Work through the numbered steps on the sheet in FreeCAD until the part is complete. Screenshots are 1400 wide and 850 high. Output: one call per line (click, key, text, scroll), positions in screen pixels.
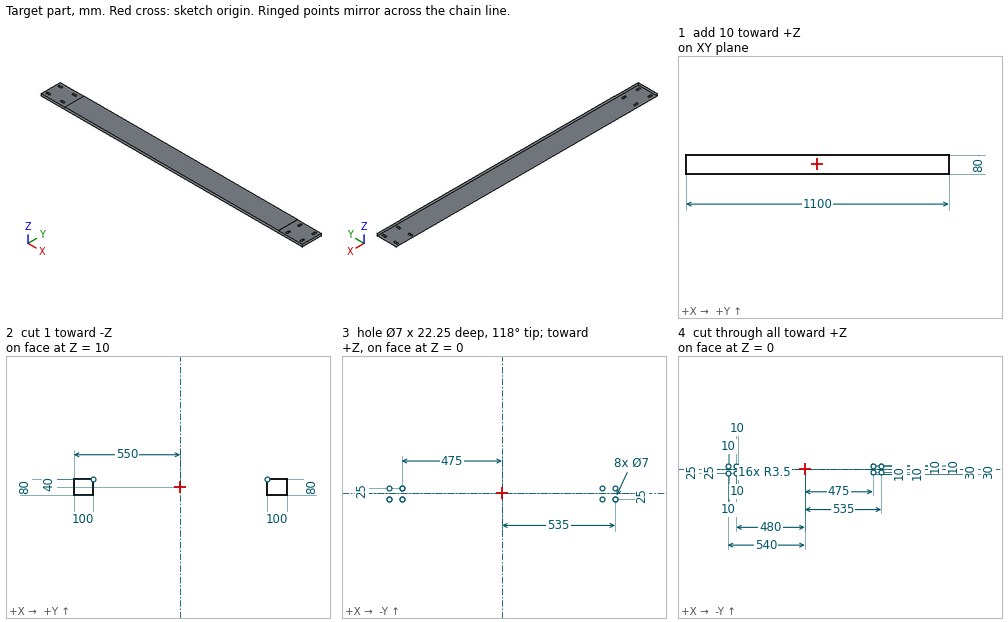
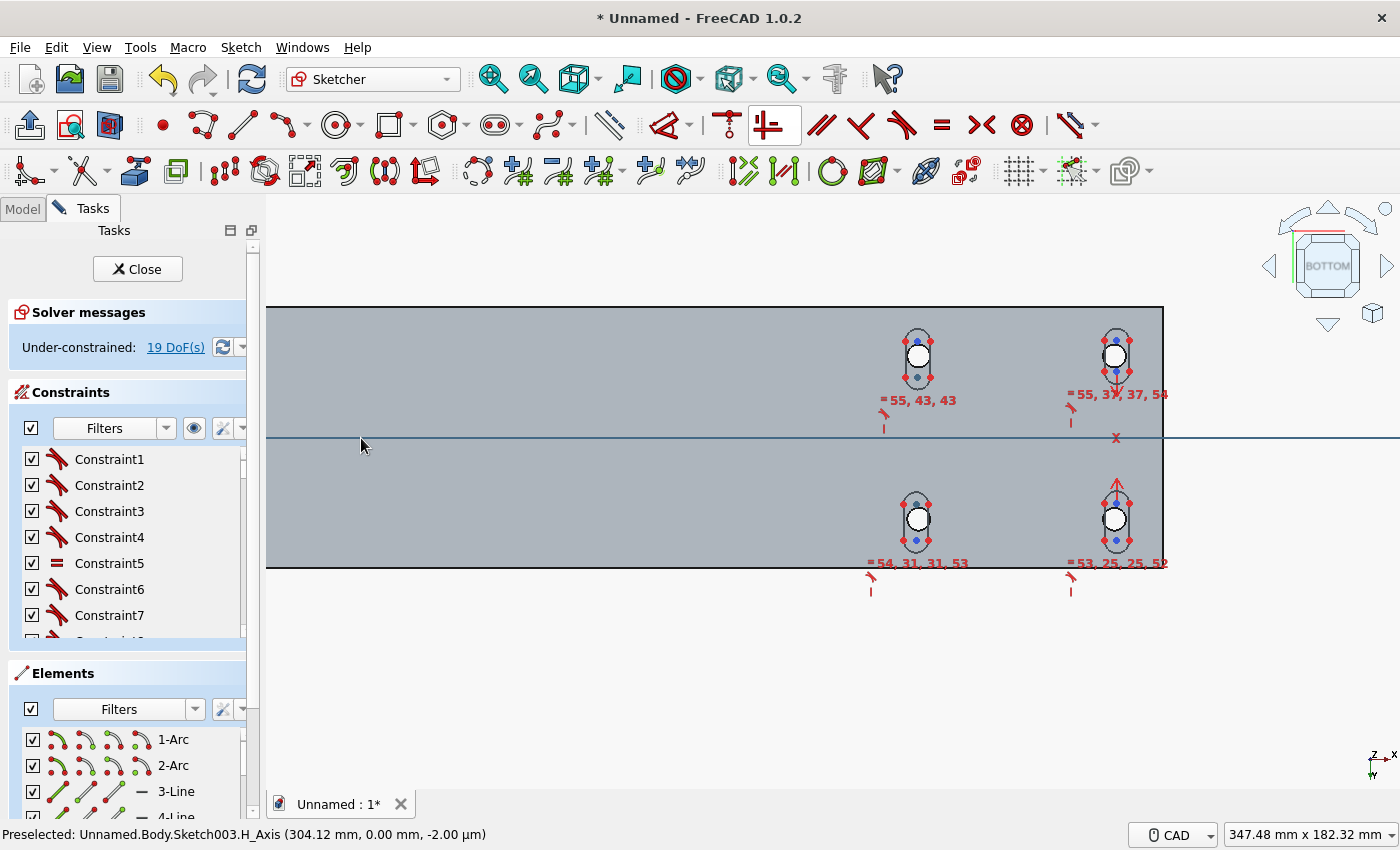
click(982, 126)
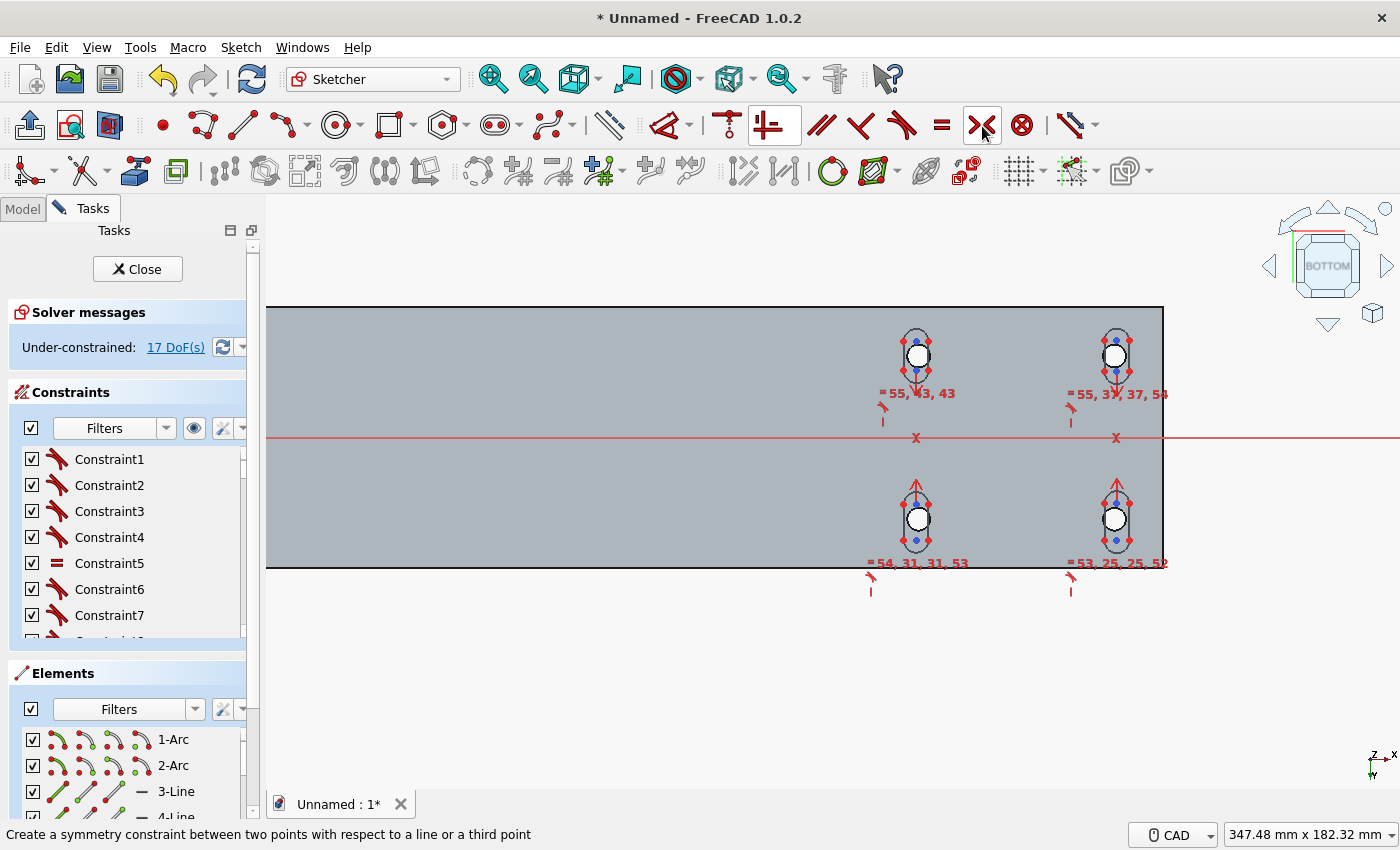
click(664, 126)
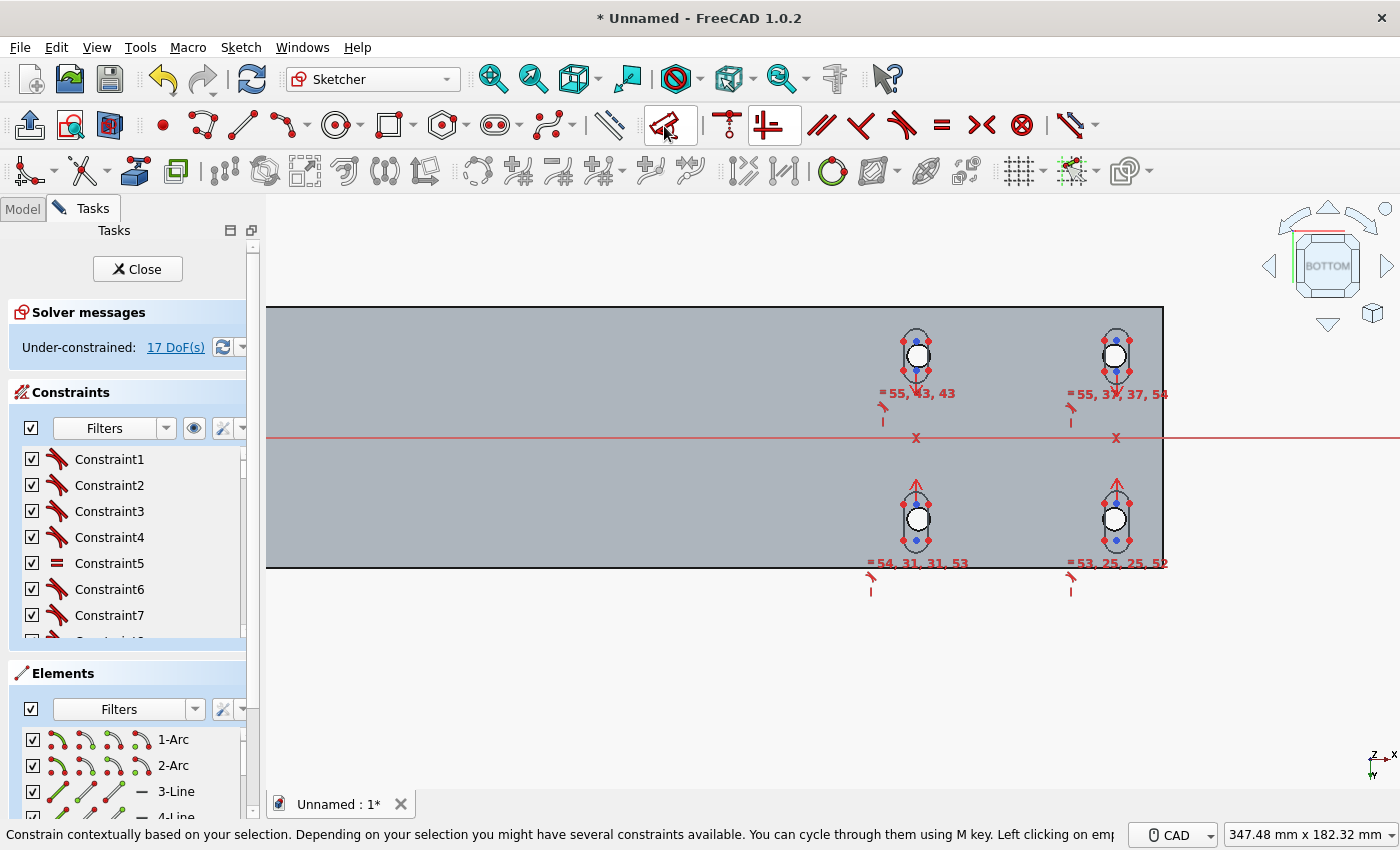
scroll(1120, 505, down, 8)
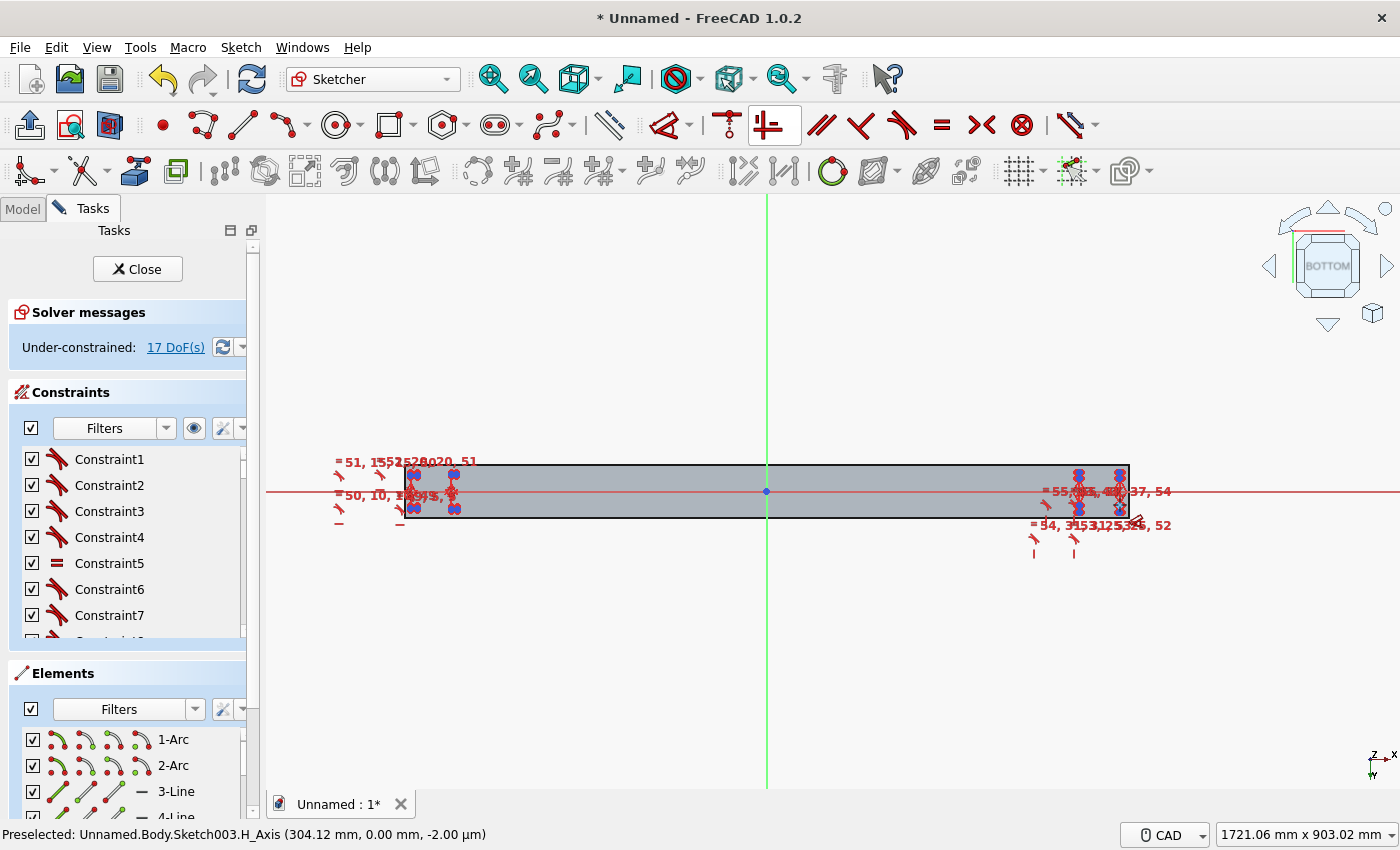
scroll(449, 508, up, 15)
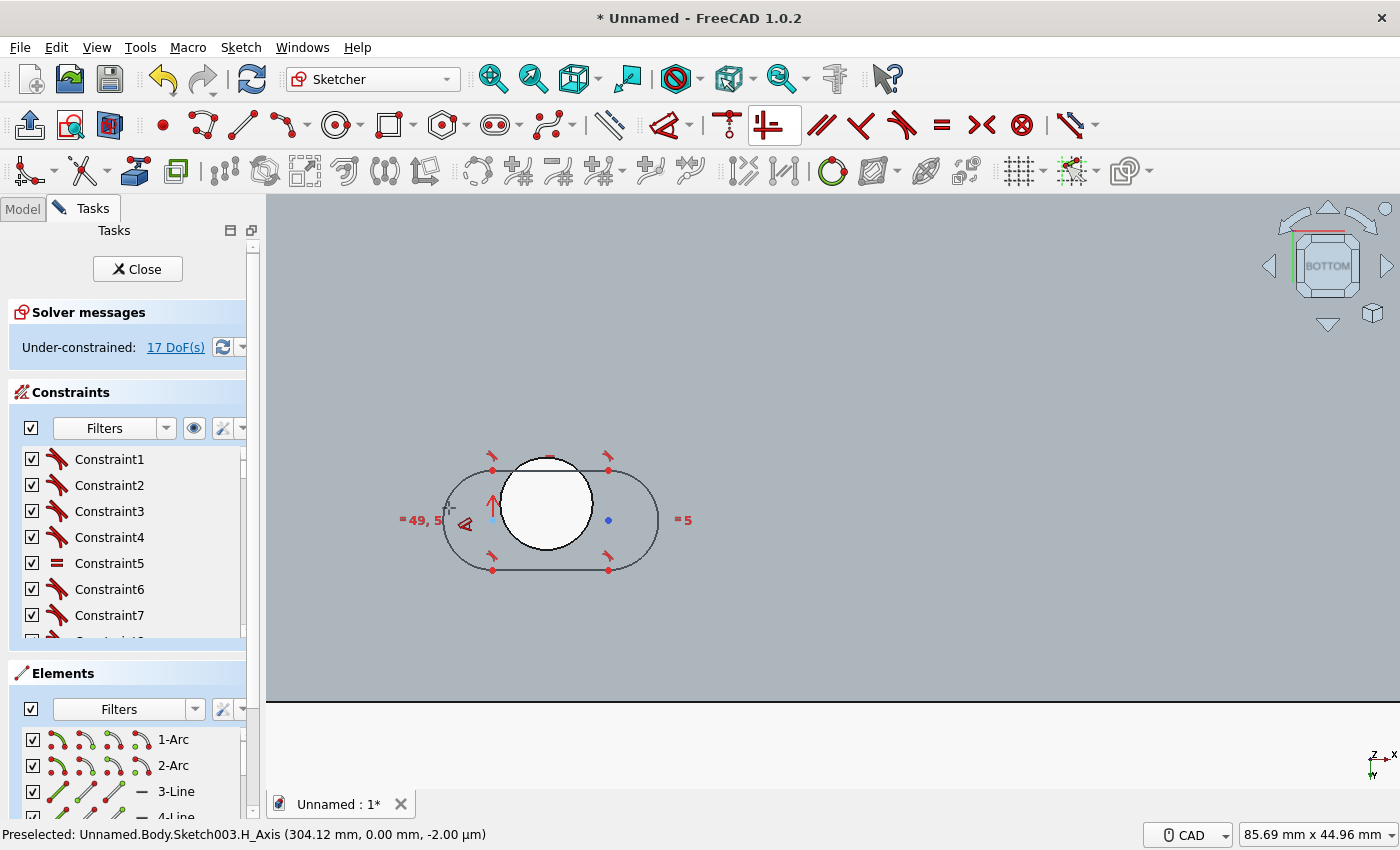
click(453, 491)
click(427, 472)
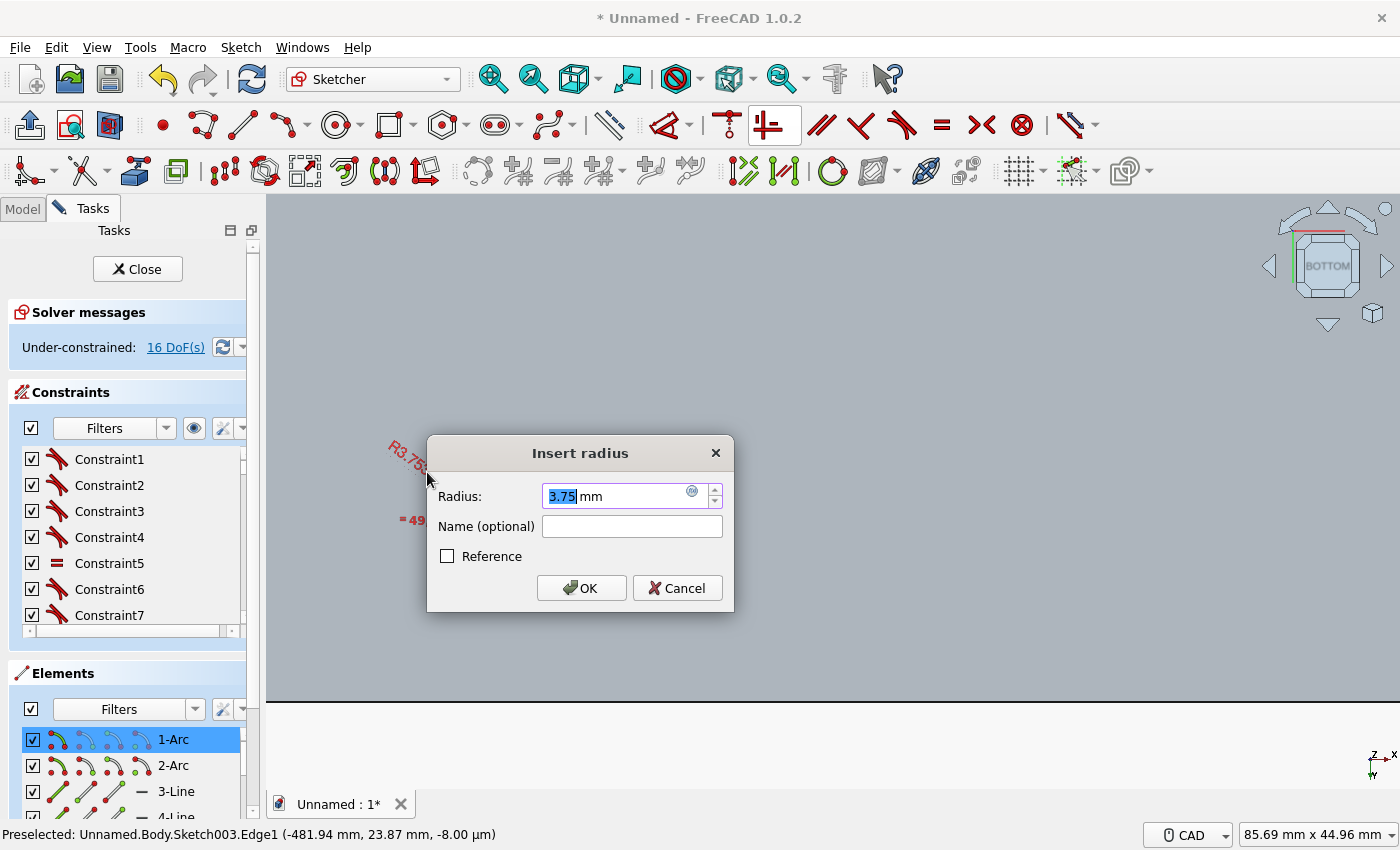
text(3.5)
key(Return)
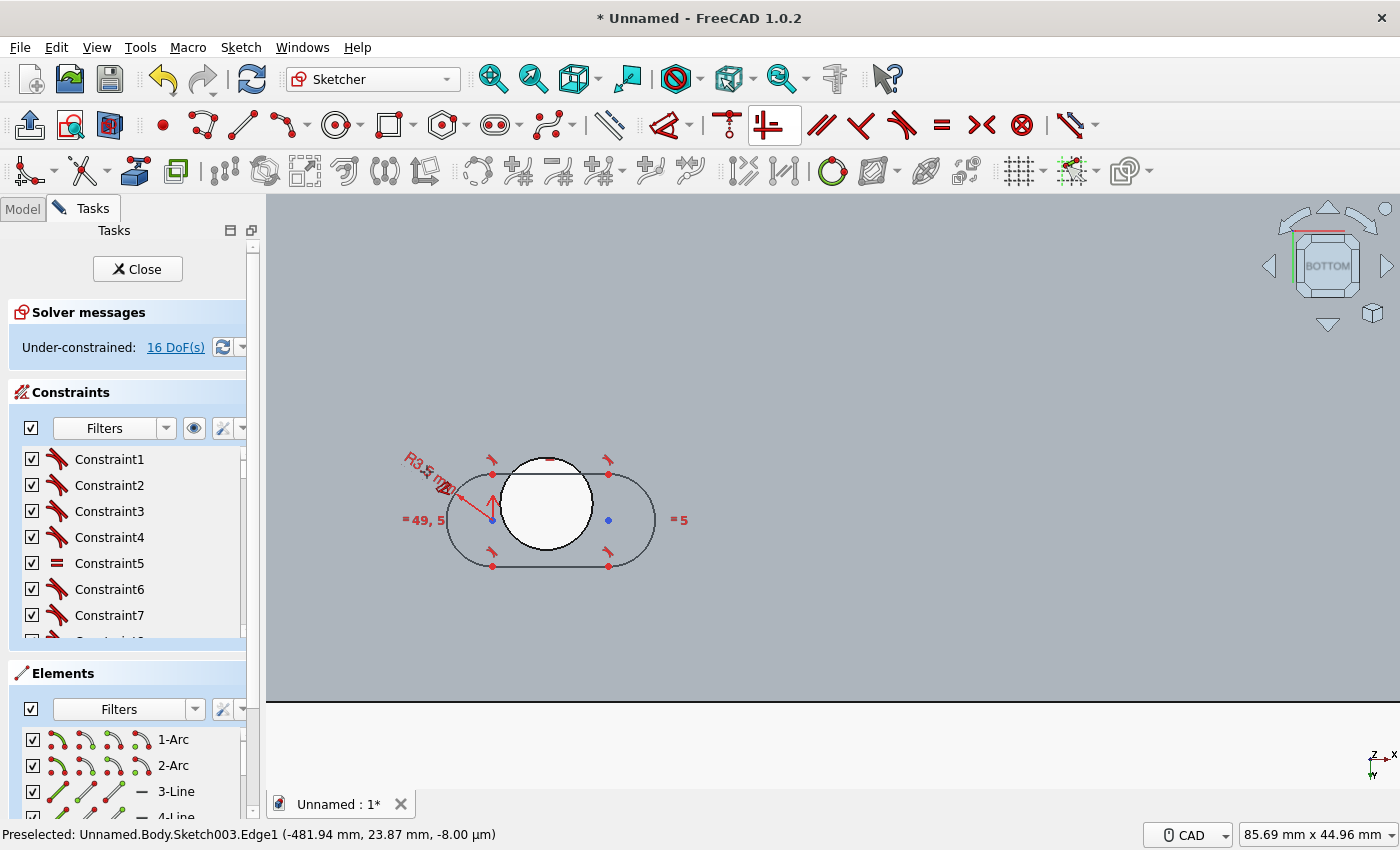
click(528, 474)
click(551, 508)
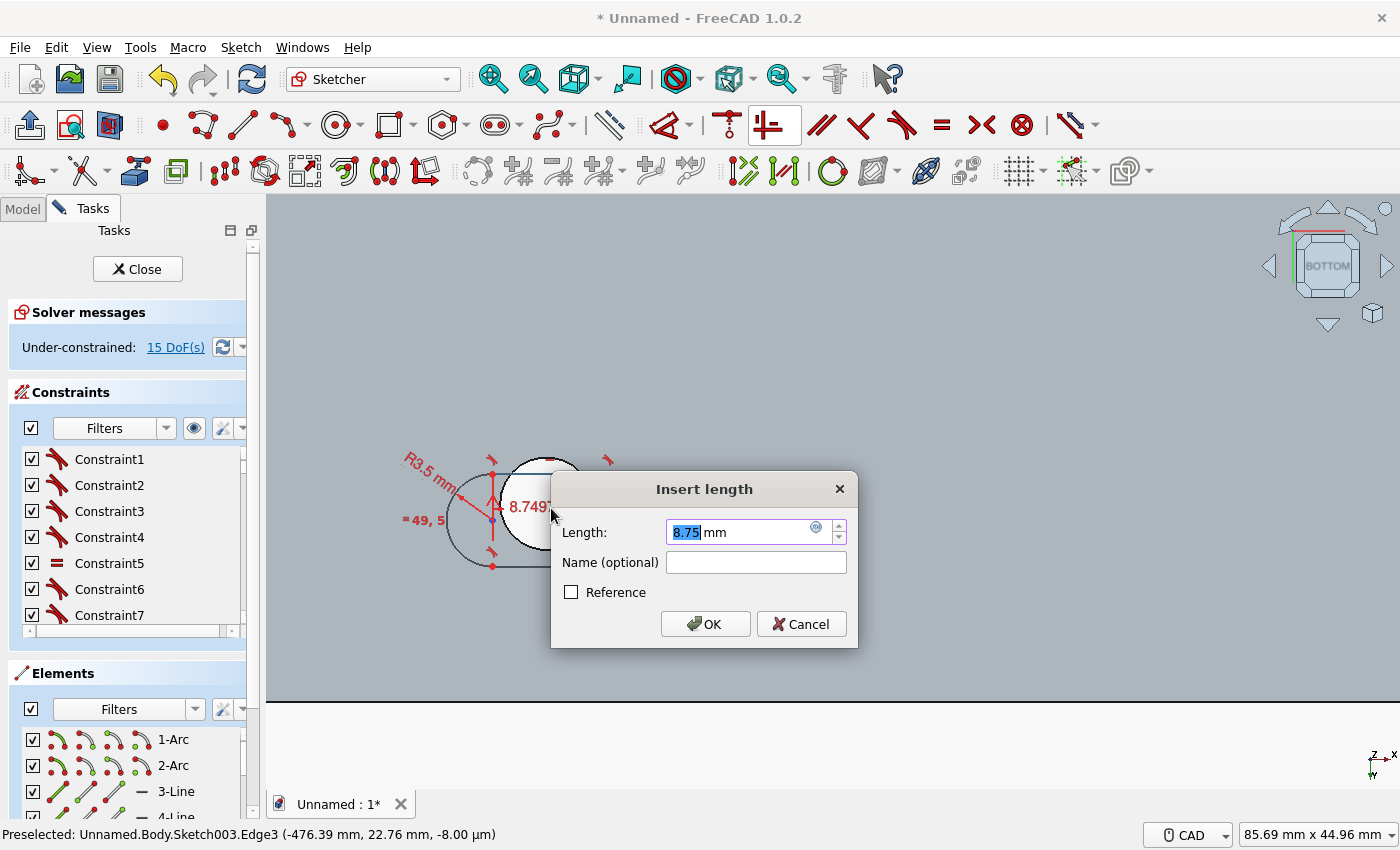
text(10)
key(Return)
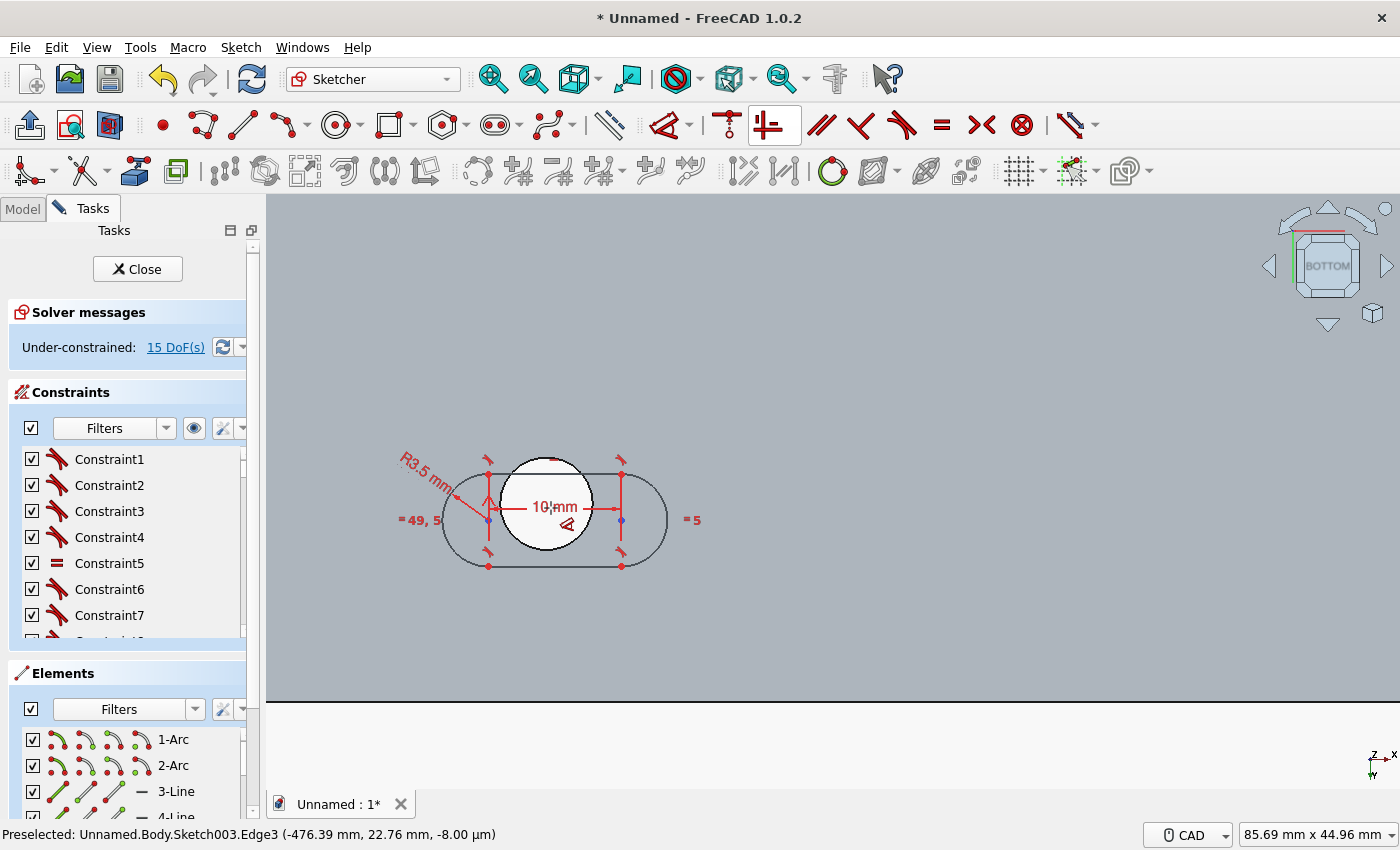
scroll(448, 508, down, 15)